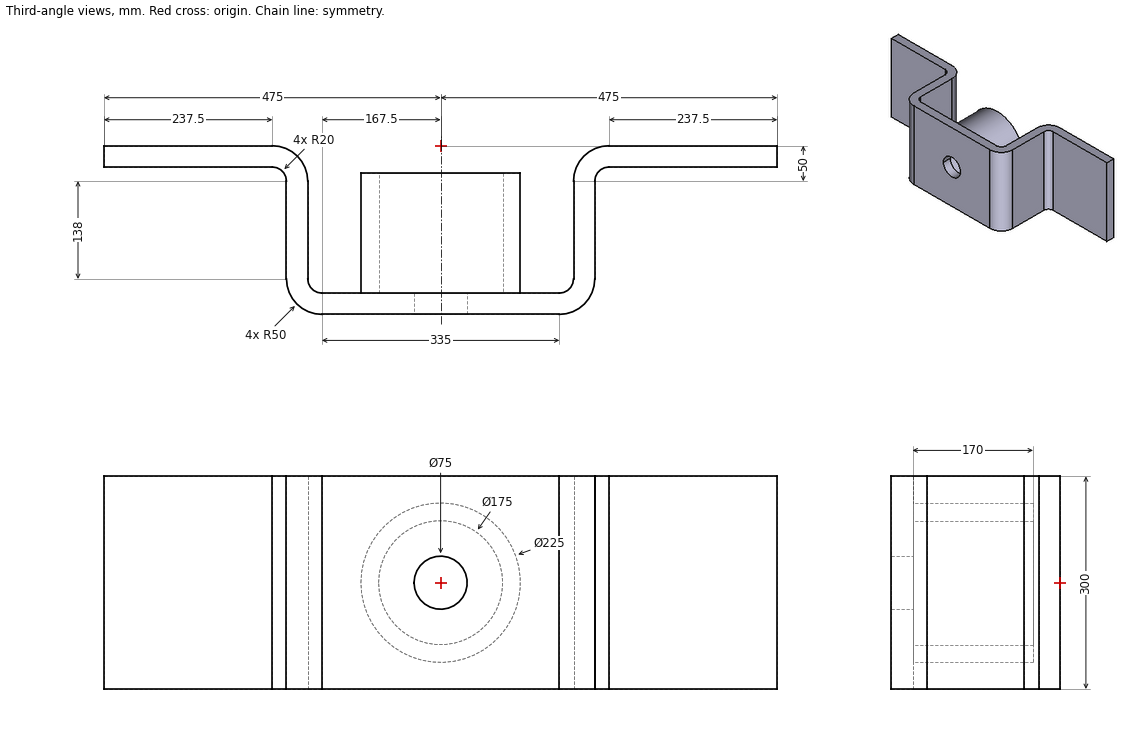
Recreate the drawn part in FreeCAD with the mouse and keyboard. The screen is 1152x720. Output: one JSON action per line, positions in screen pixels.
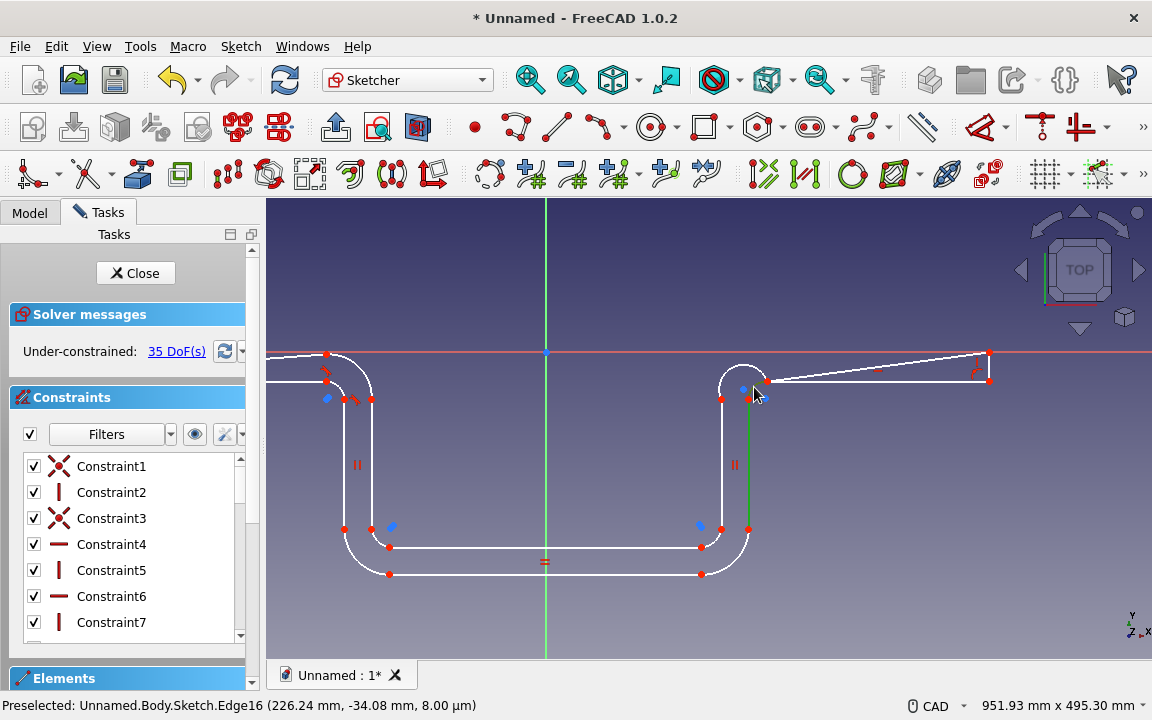
{"action": "key", "text": "t"}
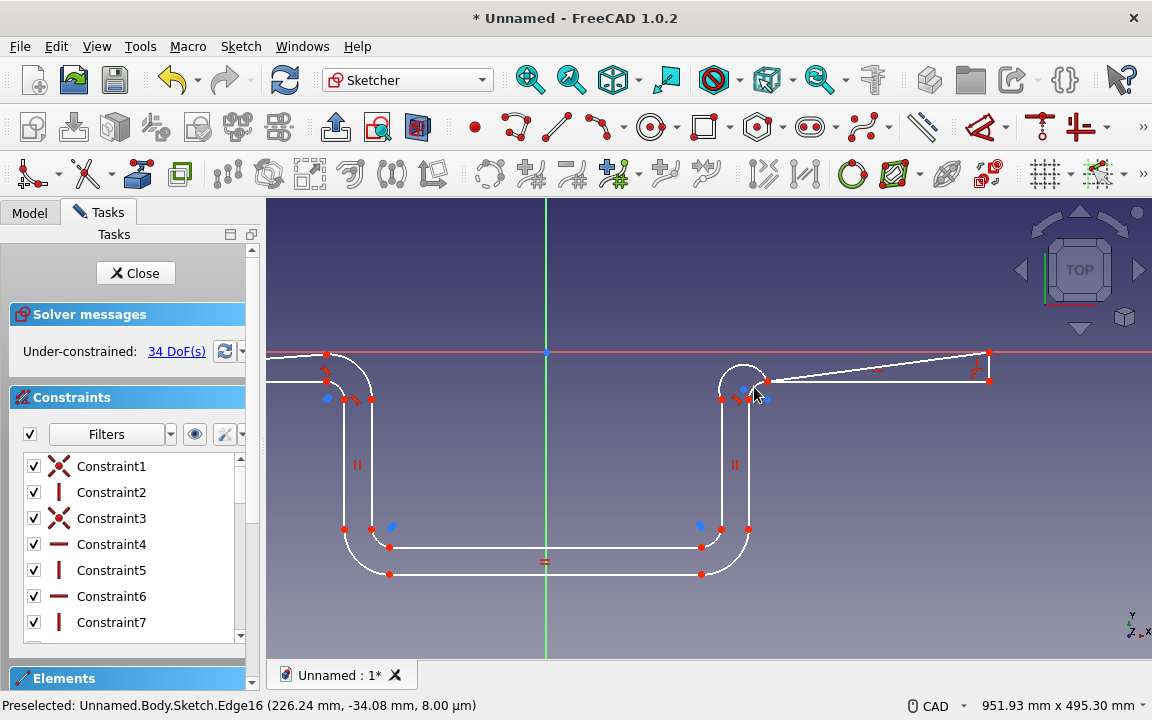
{"action": "left_click", "coordinate": [923, 382]}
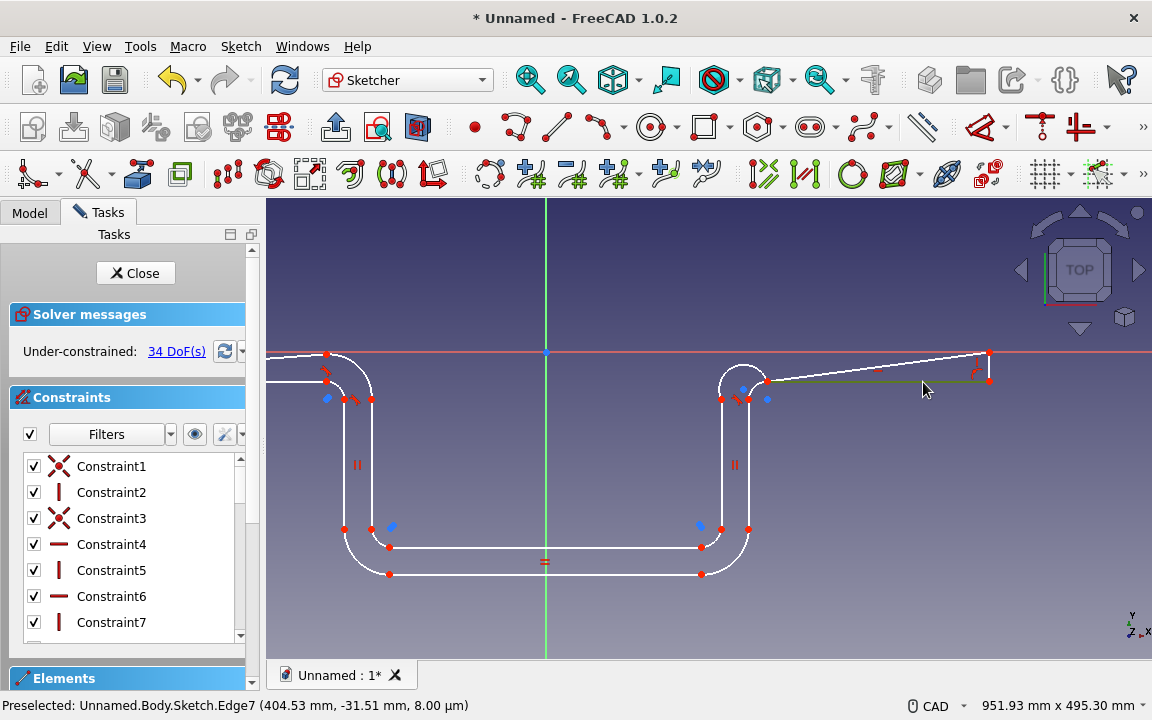
{"action": "left_click", "coordinate": [754, 387]}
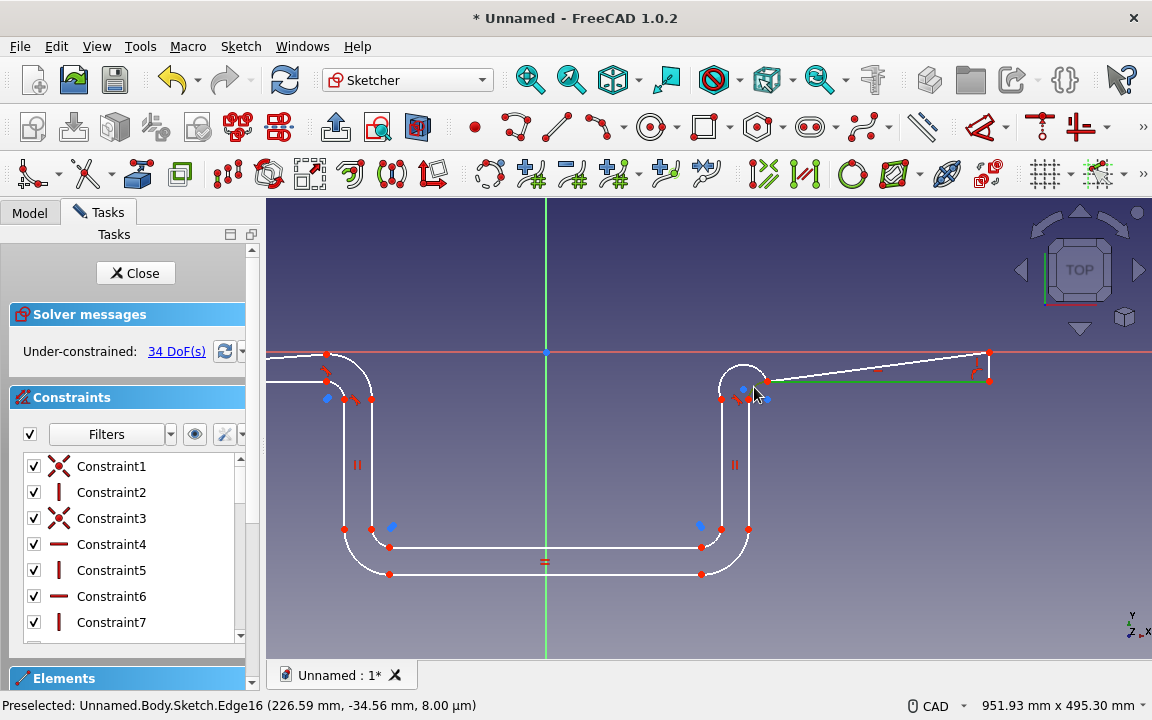
{"action": "key", "text": "t"}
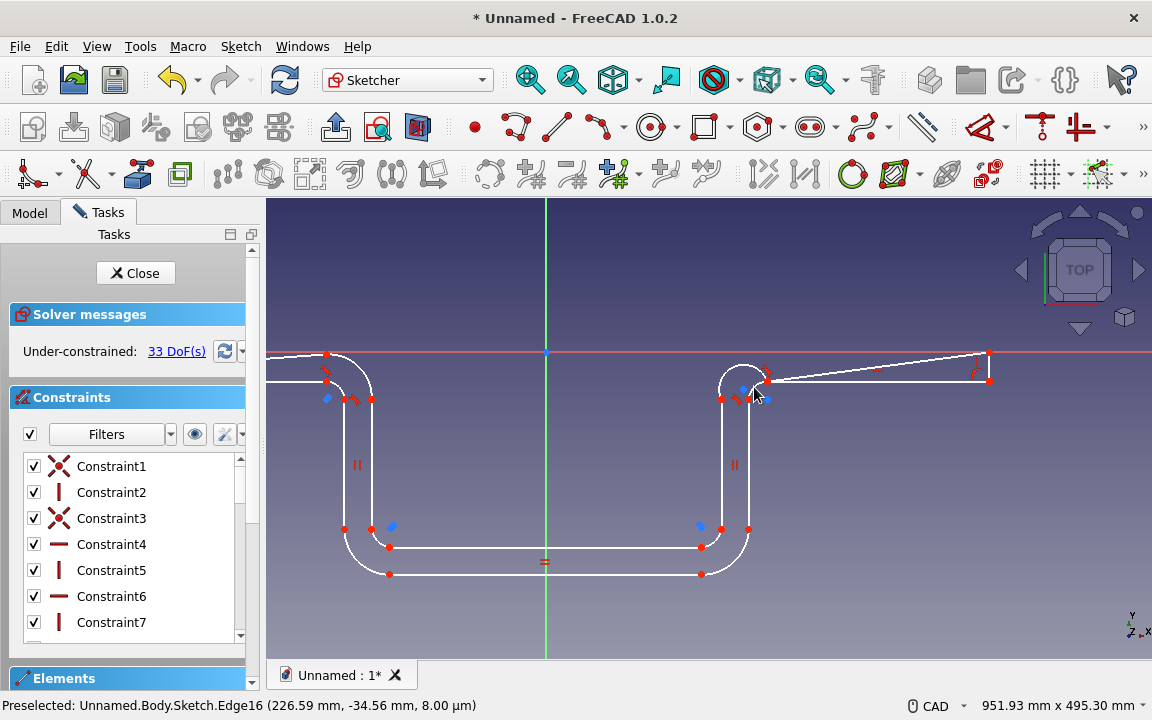
{"action": "left_click", "coordinate": [722, 439]}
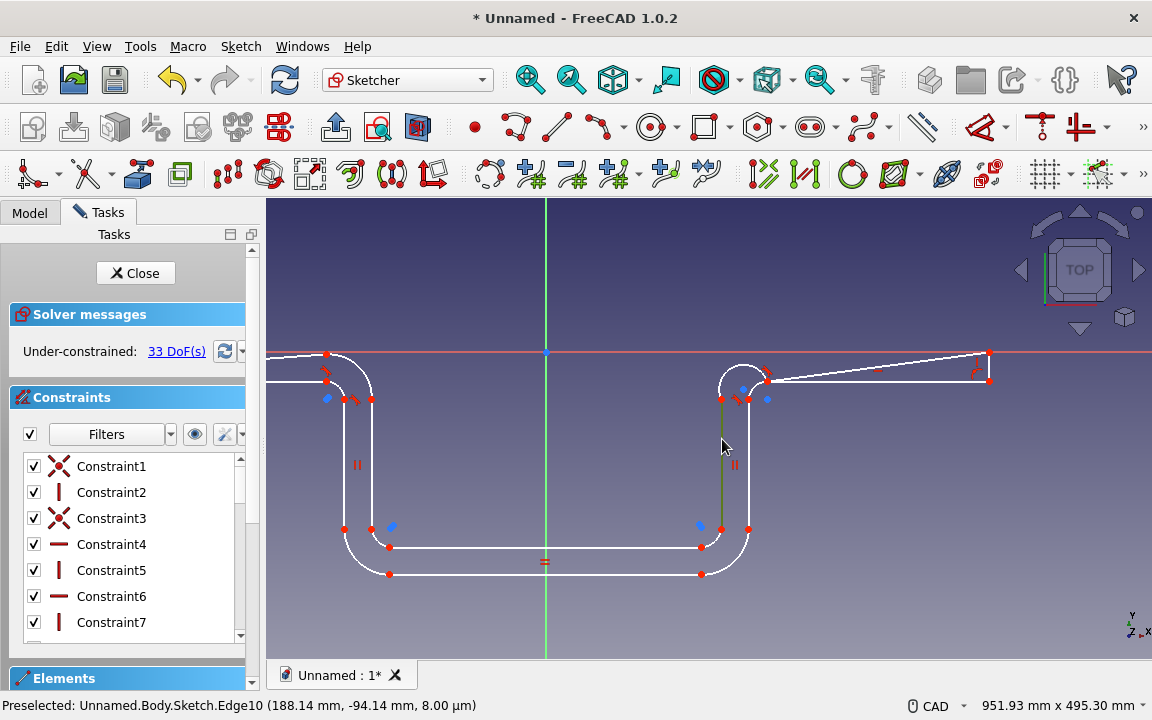
{"action": "left_click", "coordinate": [715, 542]}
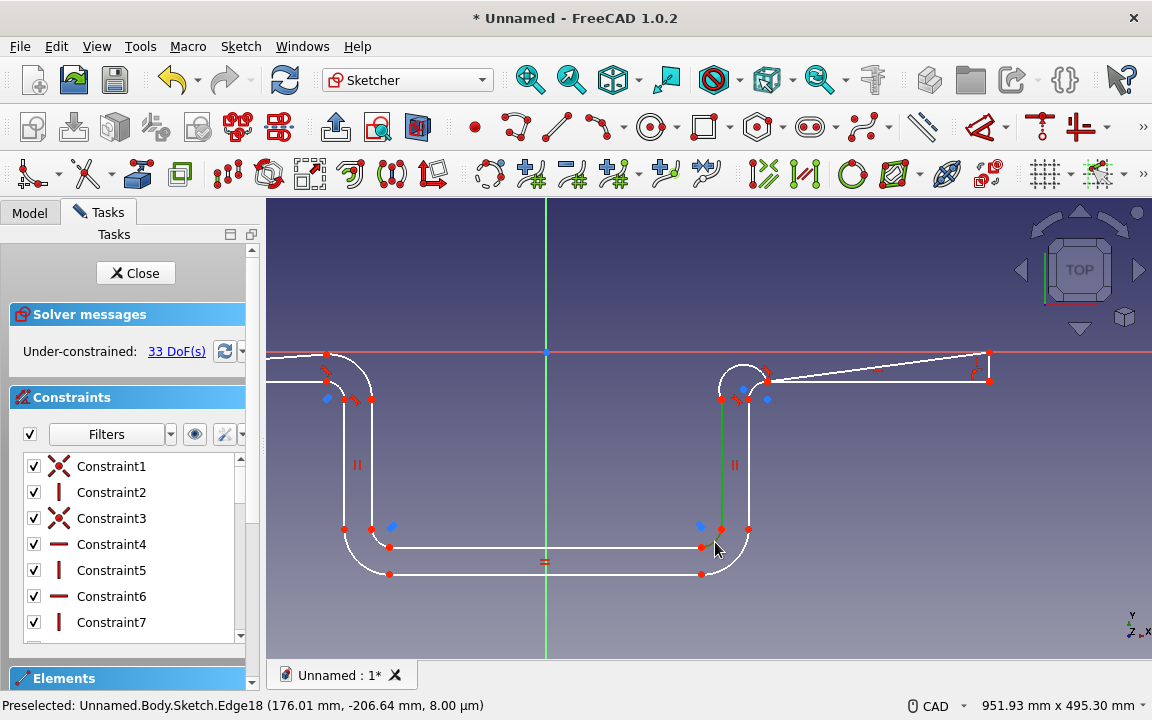
{"action": "key", "text": "t"}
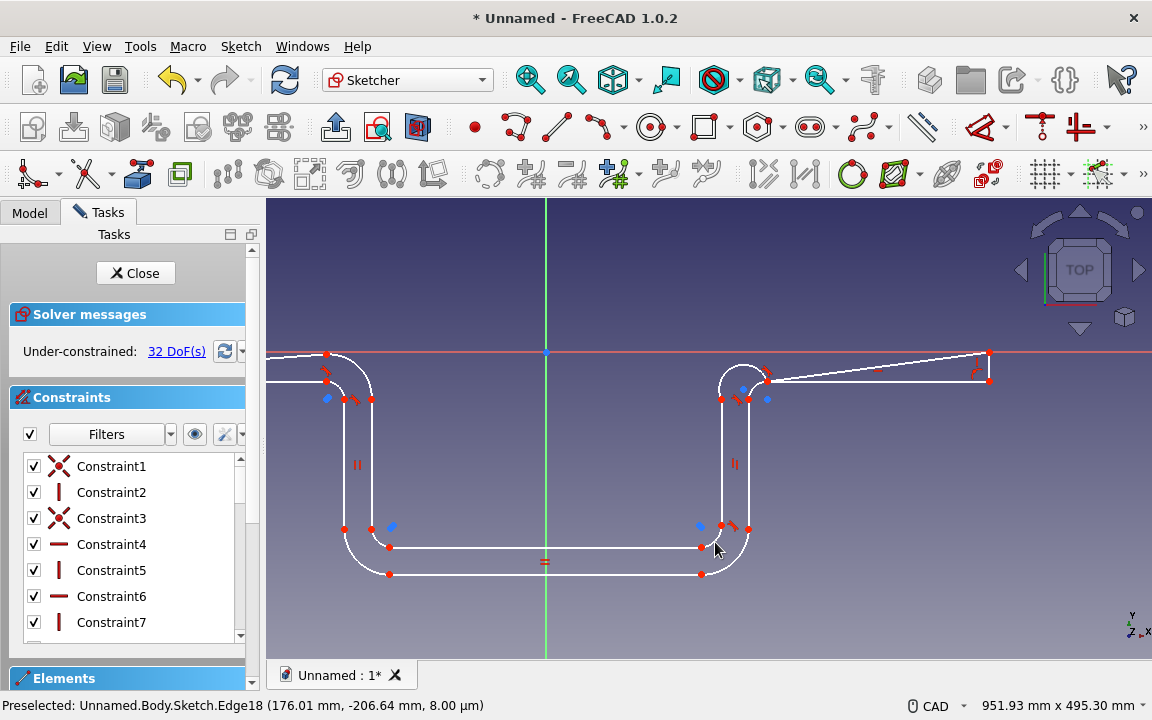
{"action": "left_click", "coordinate": [608, 548]}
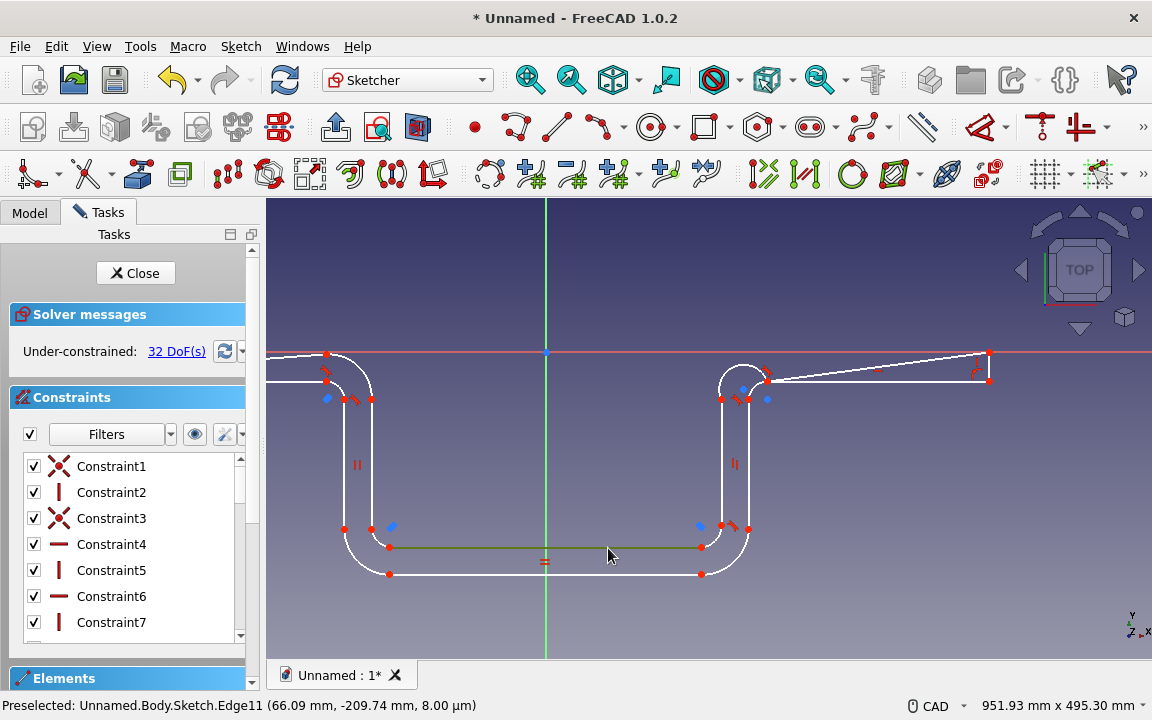
{"action": "scroll", "coordinate": [711, 544], "scroll_direction": "up", "scroll_amount": 2}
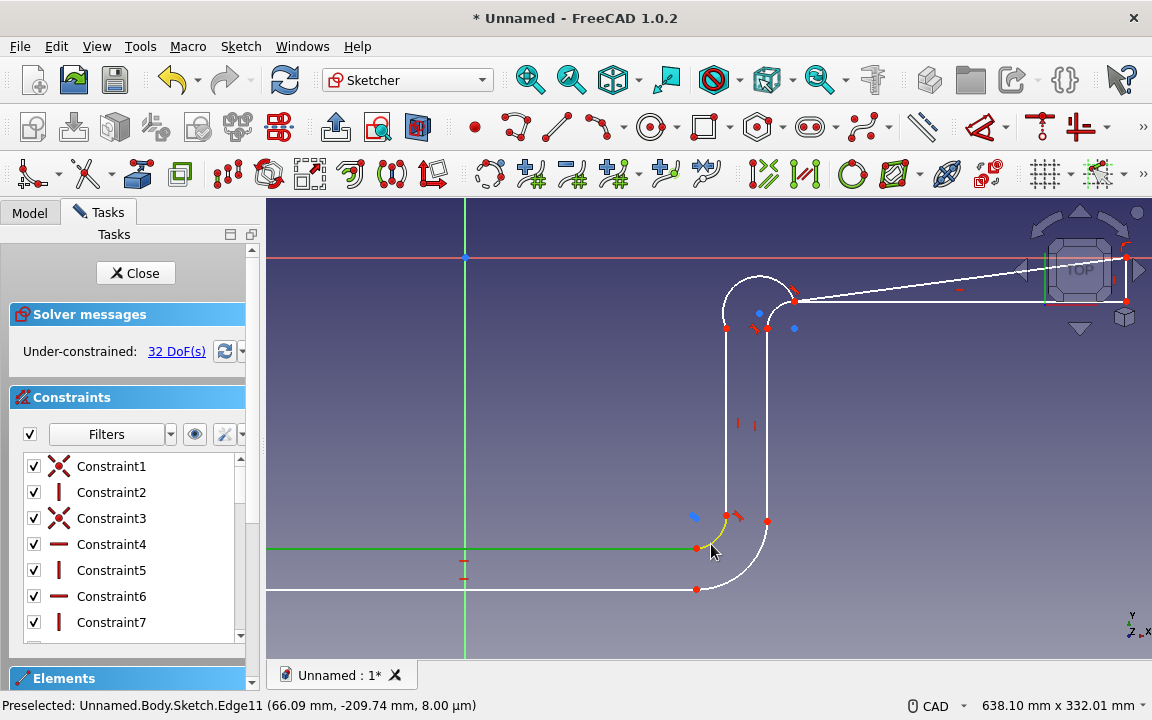
{"action": "left_click", "coordinate": [710, 544]}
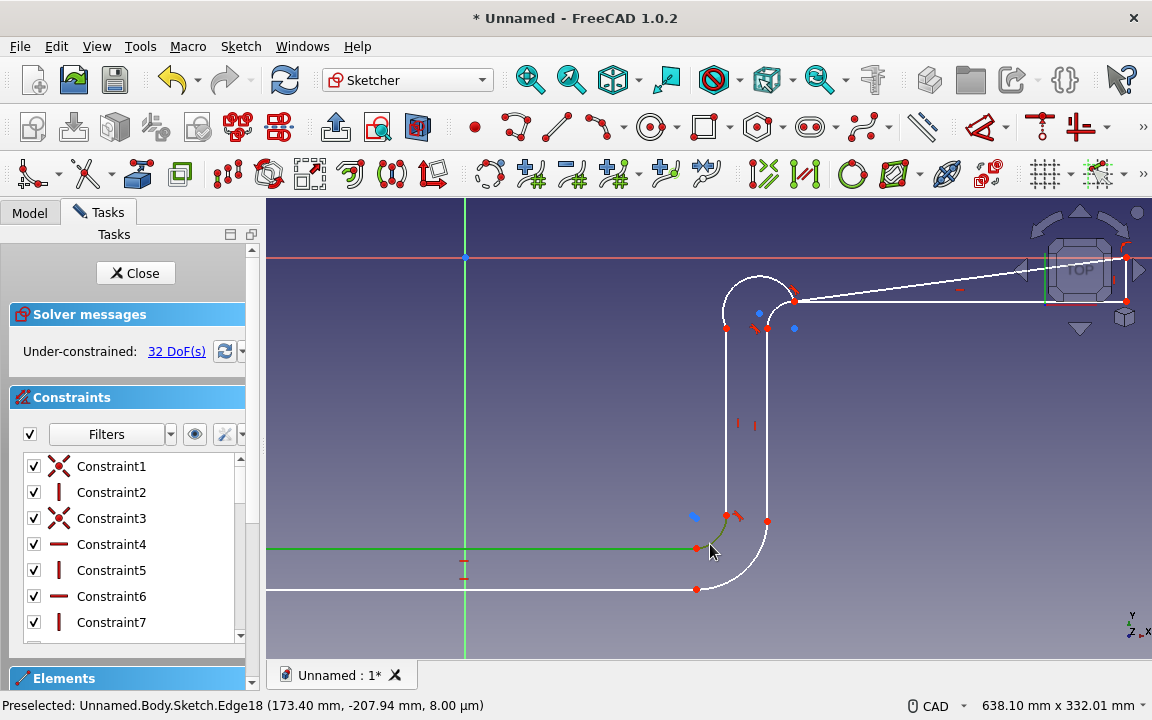
{"action": "key", "text": "t"}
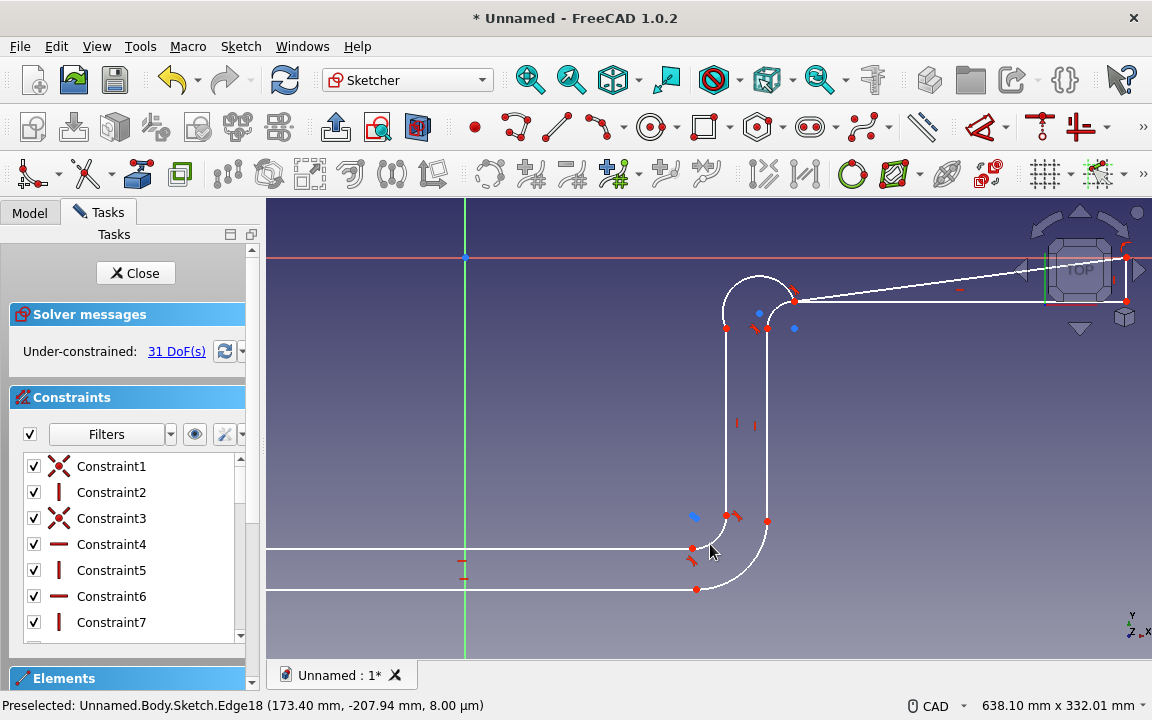
{"action": "left_click", "coordinate": [555, 549]}